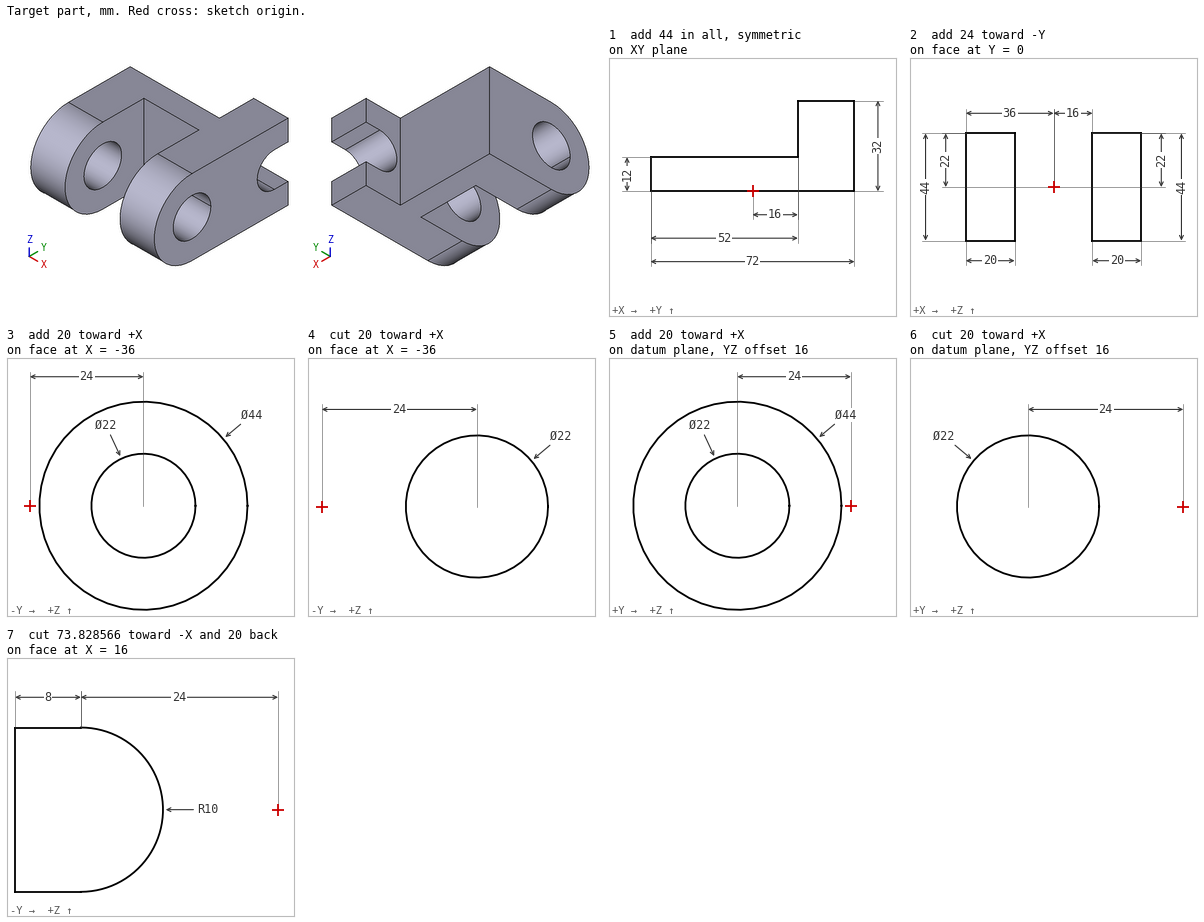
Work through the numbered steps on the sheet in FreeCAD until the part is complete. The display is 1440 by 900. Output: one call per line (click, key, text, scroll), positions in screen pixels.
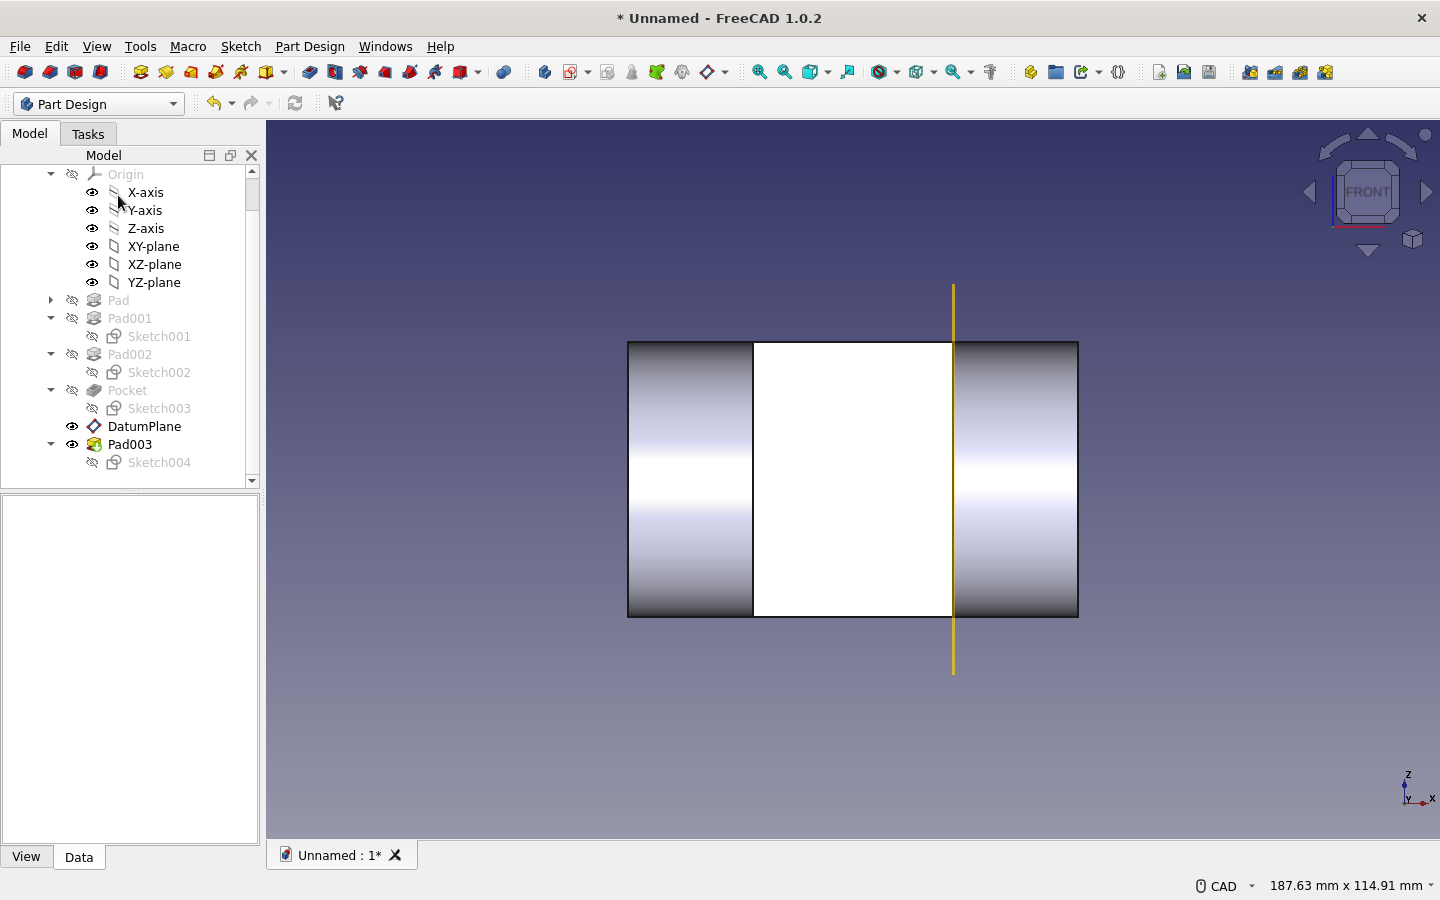
click(117, 426)
key(space)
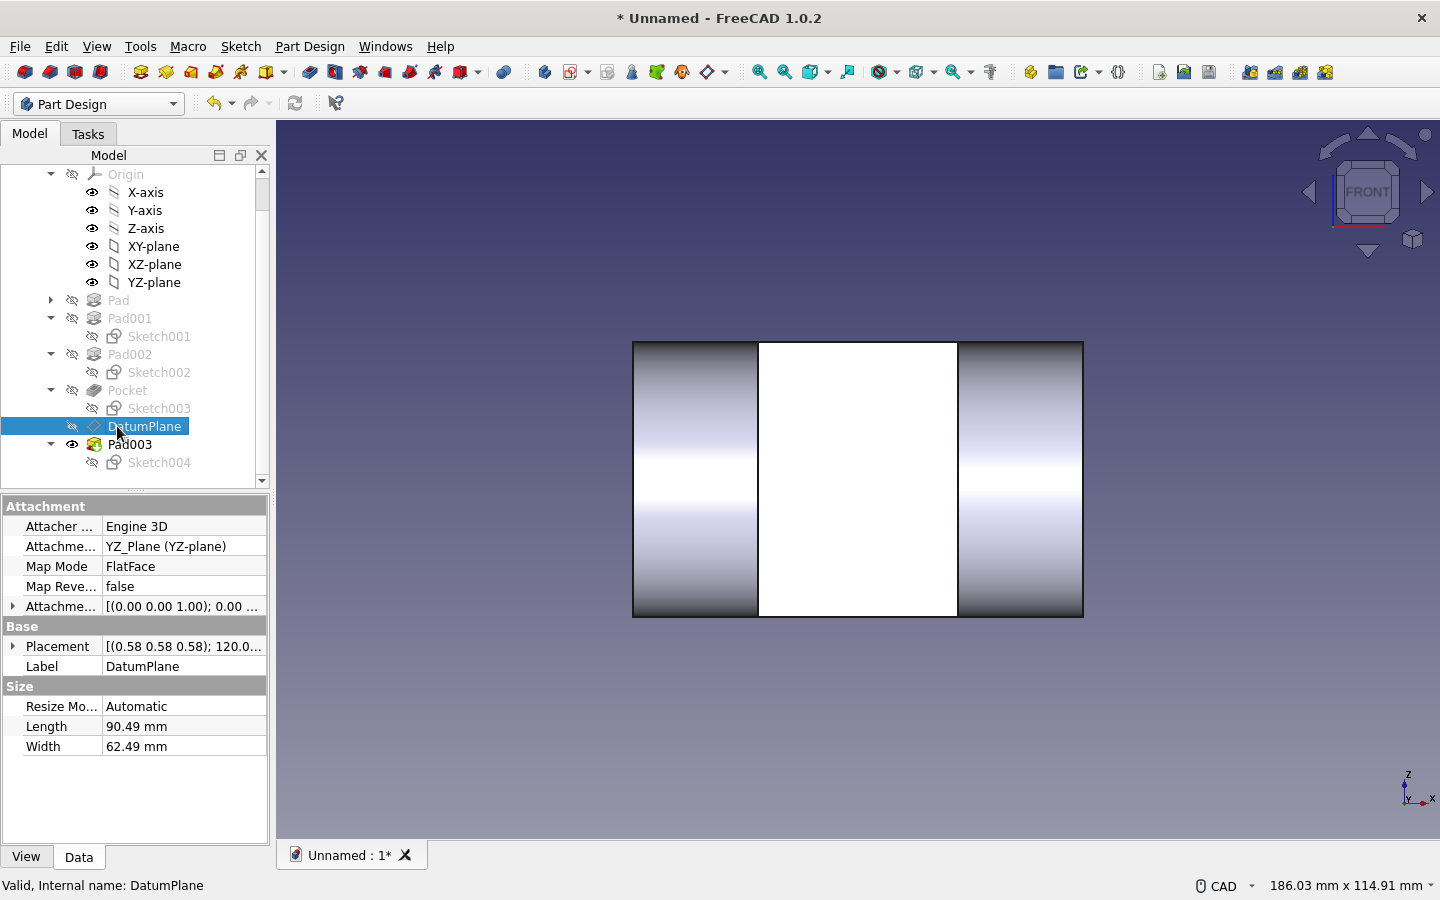
click(760, 72)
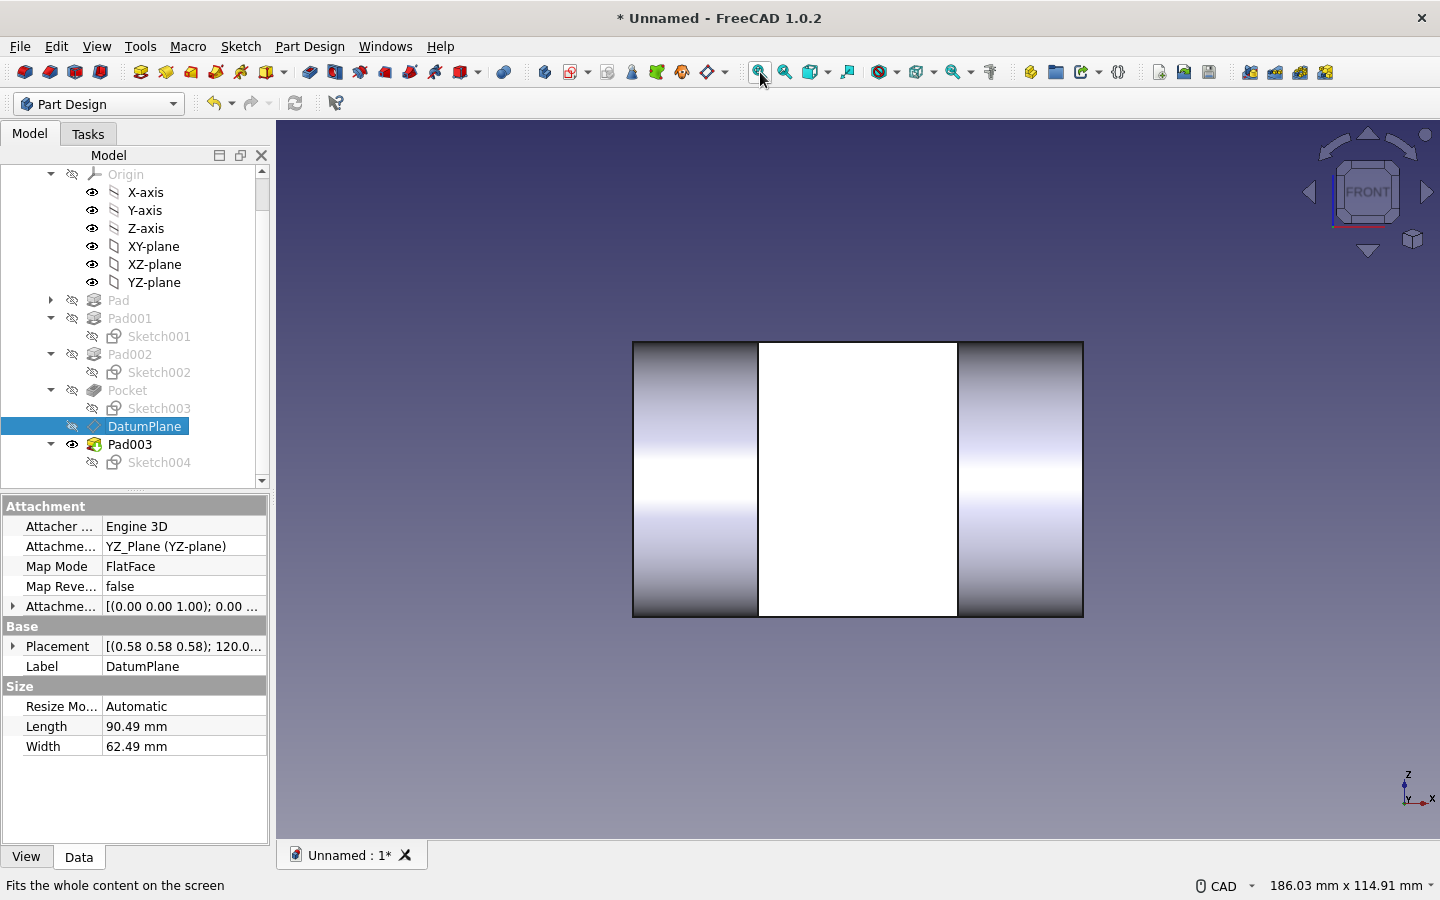
key(6)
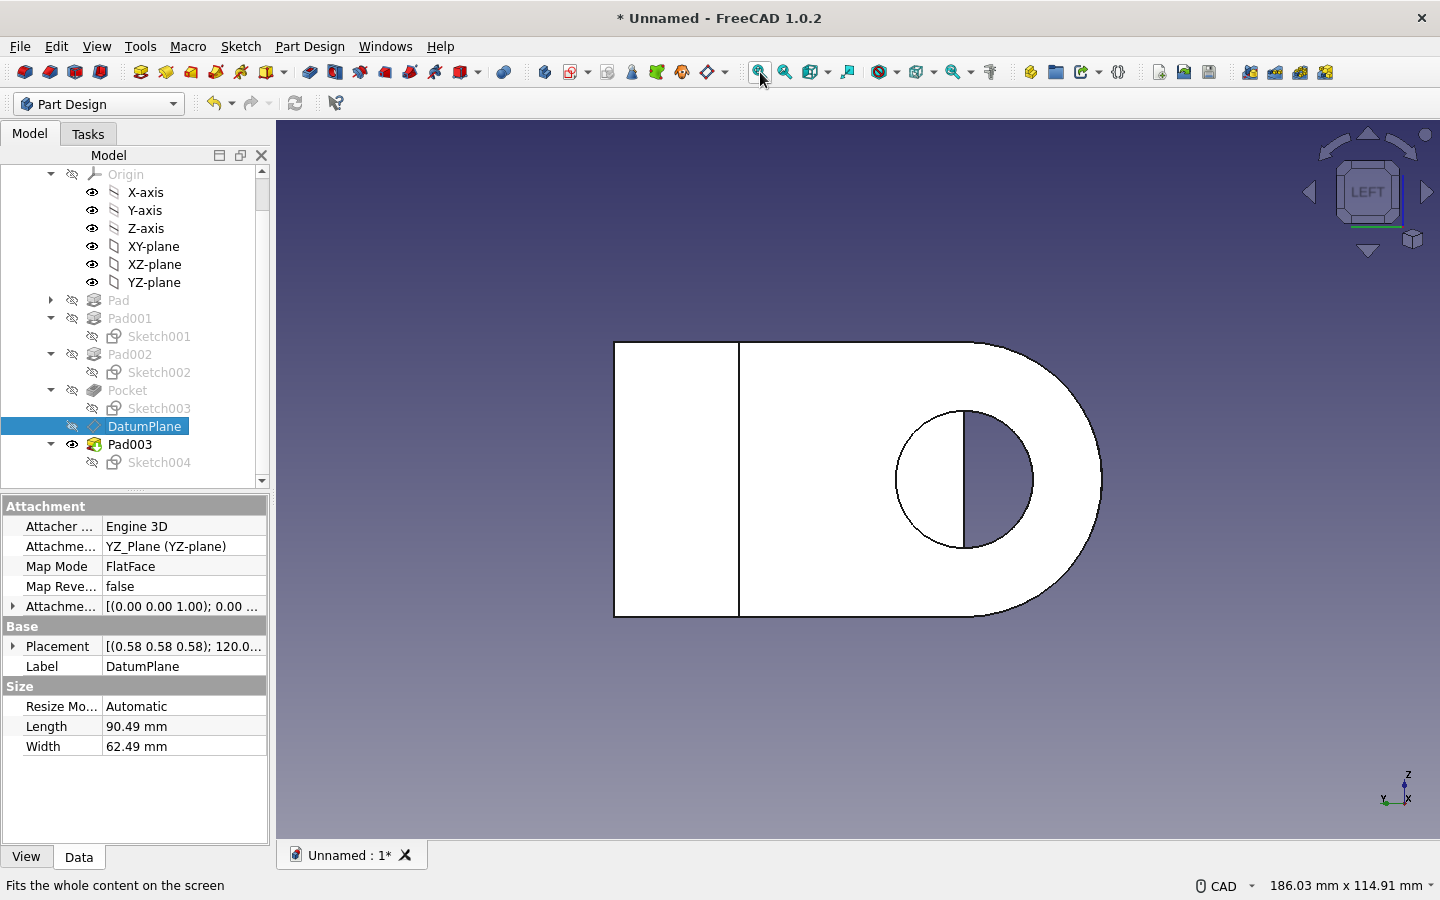
click(760, 72)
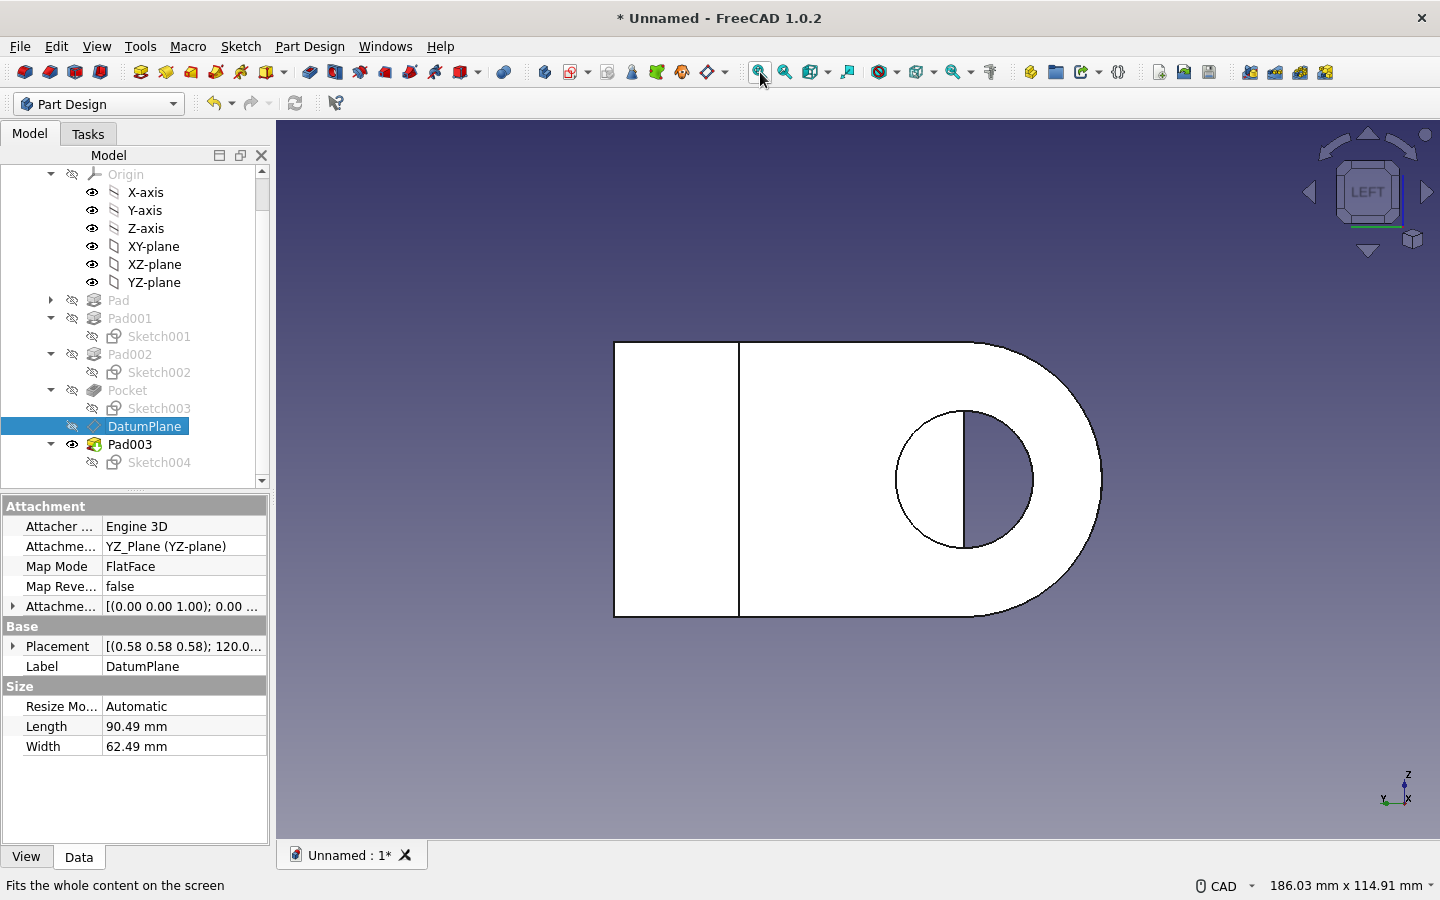
key(2)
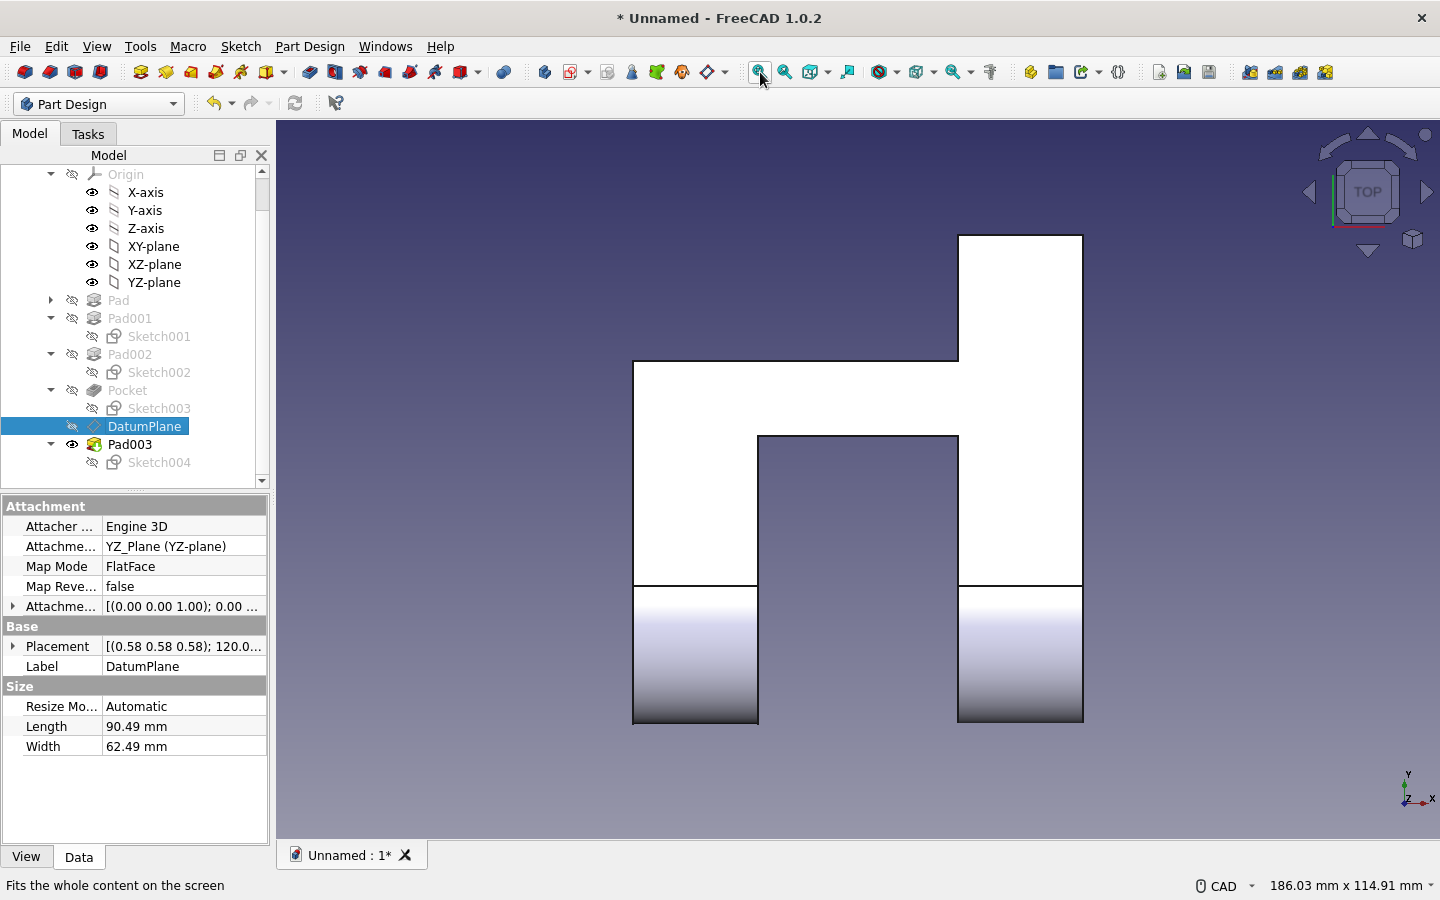
key(1)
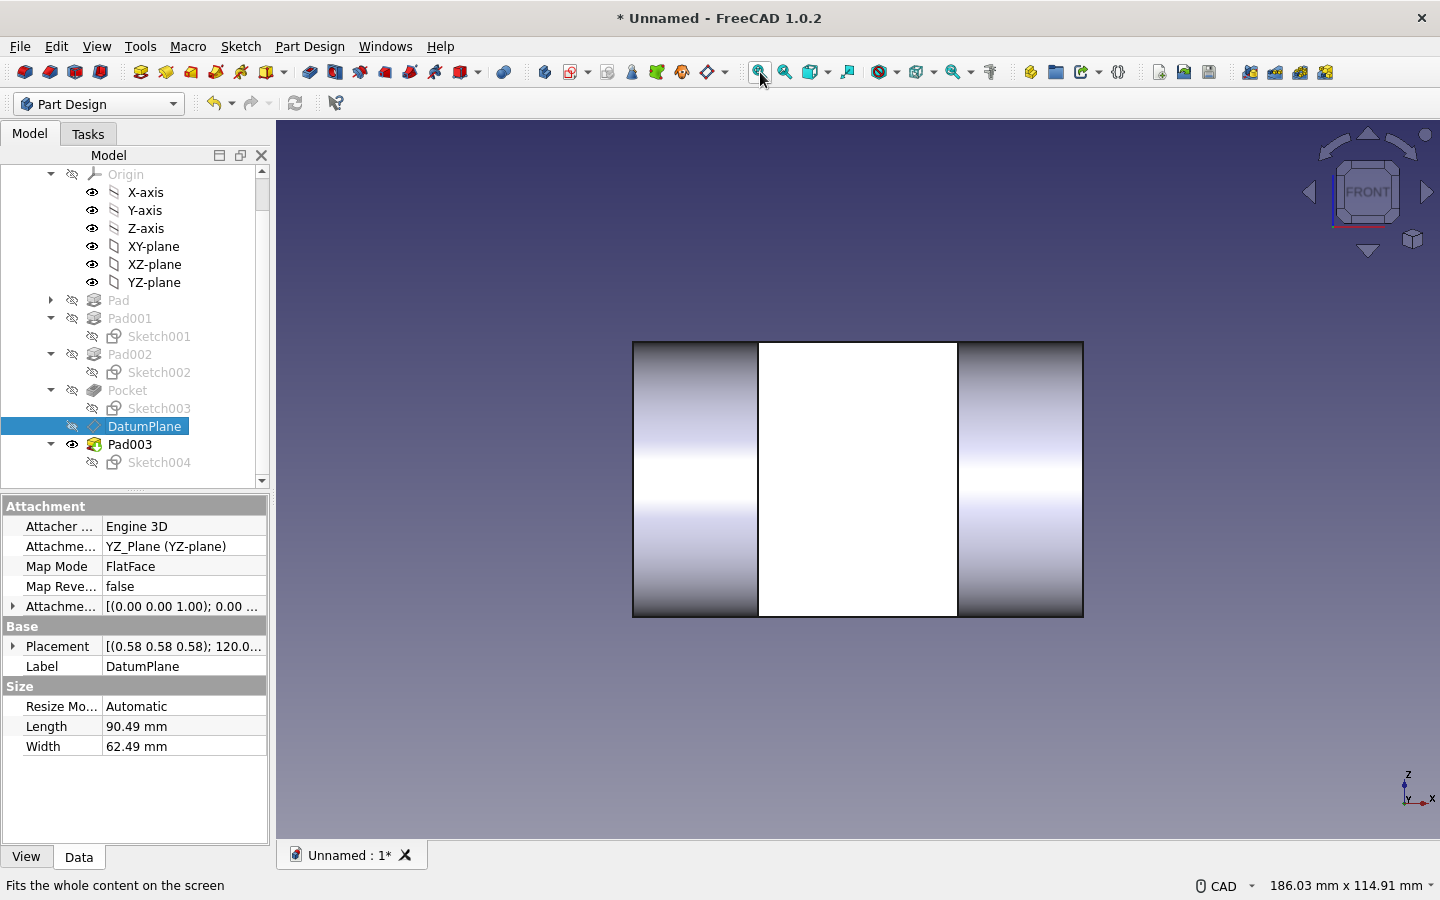
click(760, 72)